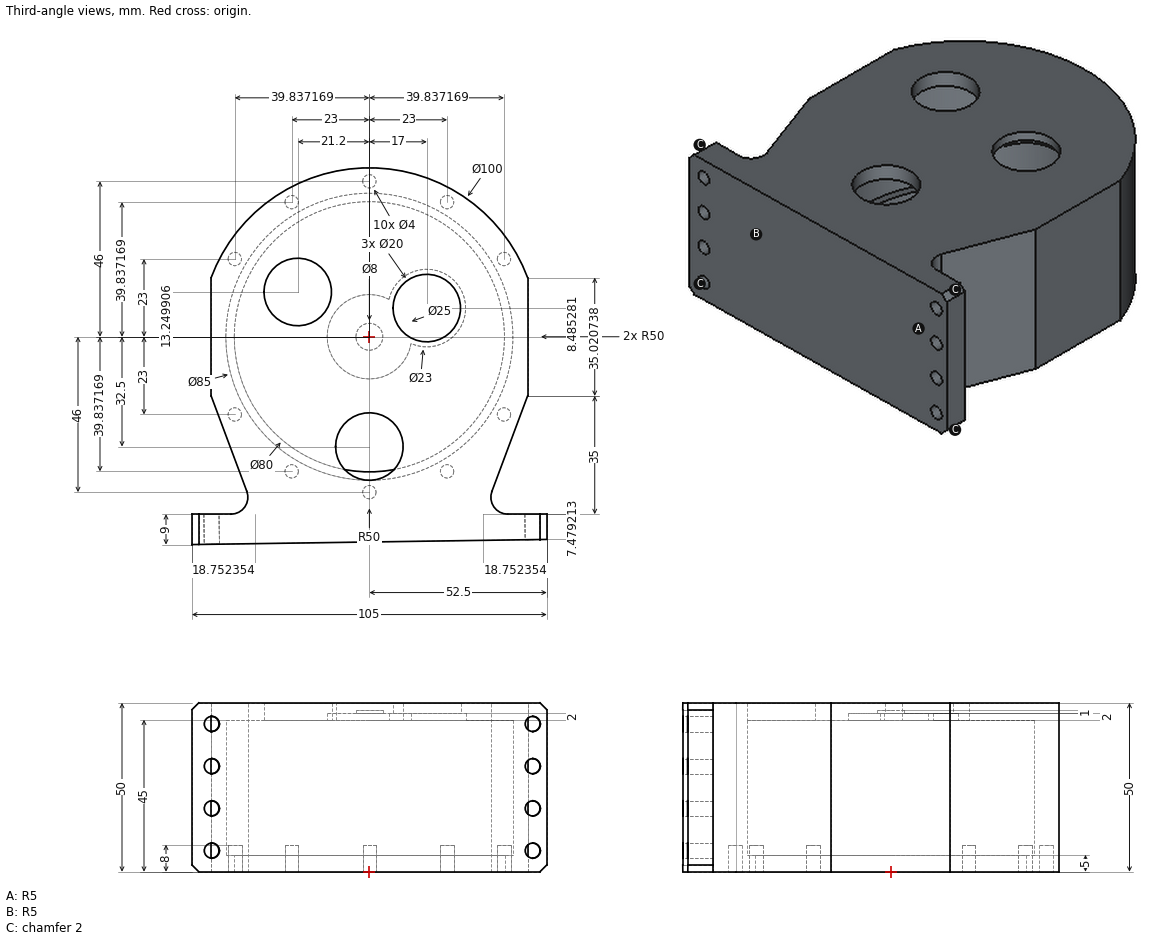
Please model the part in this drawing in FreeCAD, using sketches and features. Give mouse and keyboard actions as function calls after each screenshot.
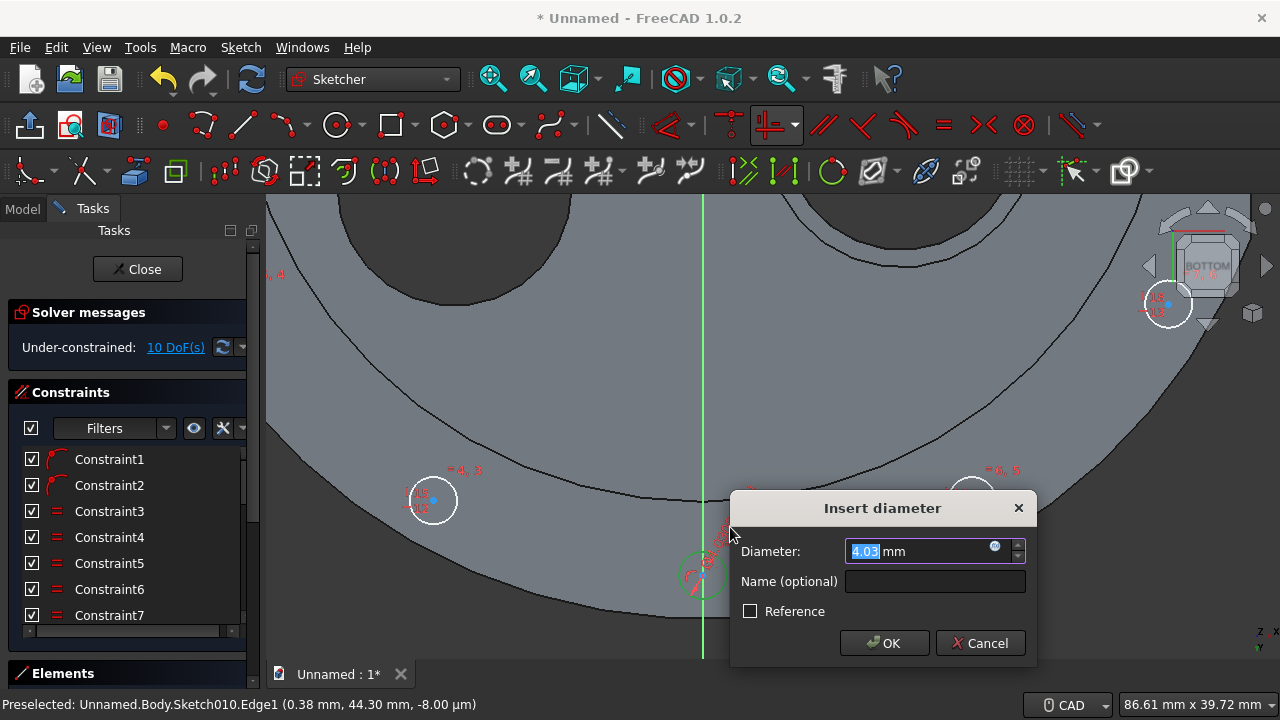
text(4)
key(Return)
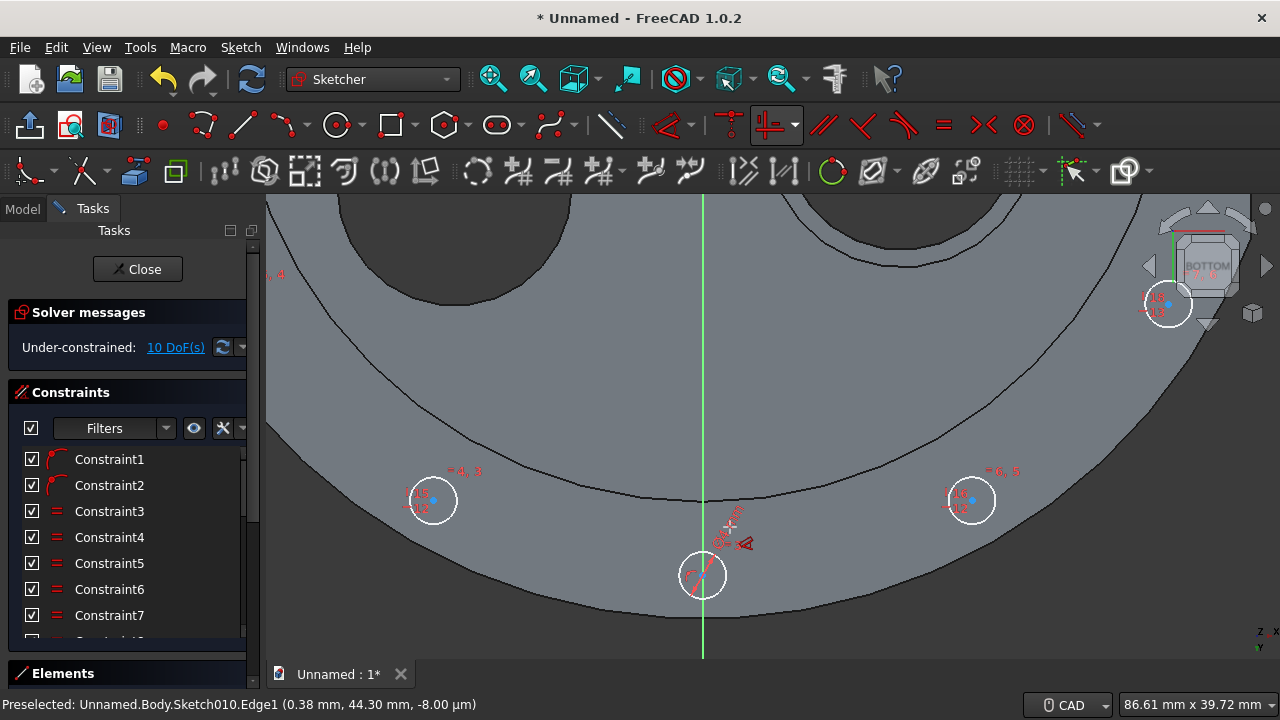
scroll(705, 555, down, 7)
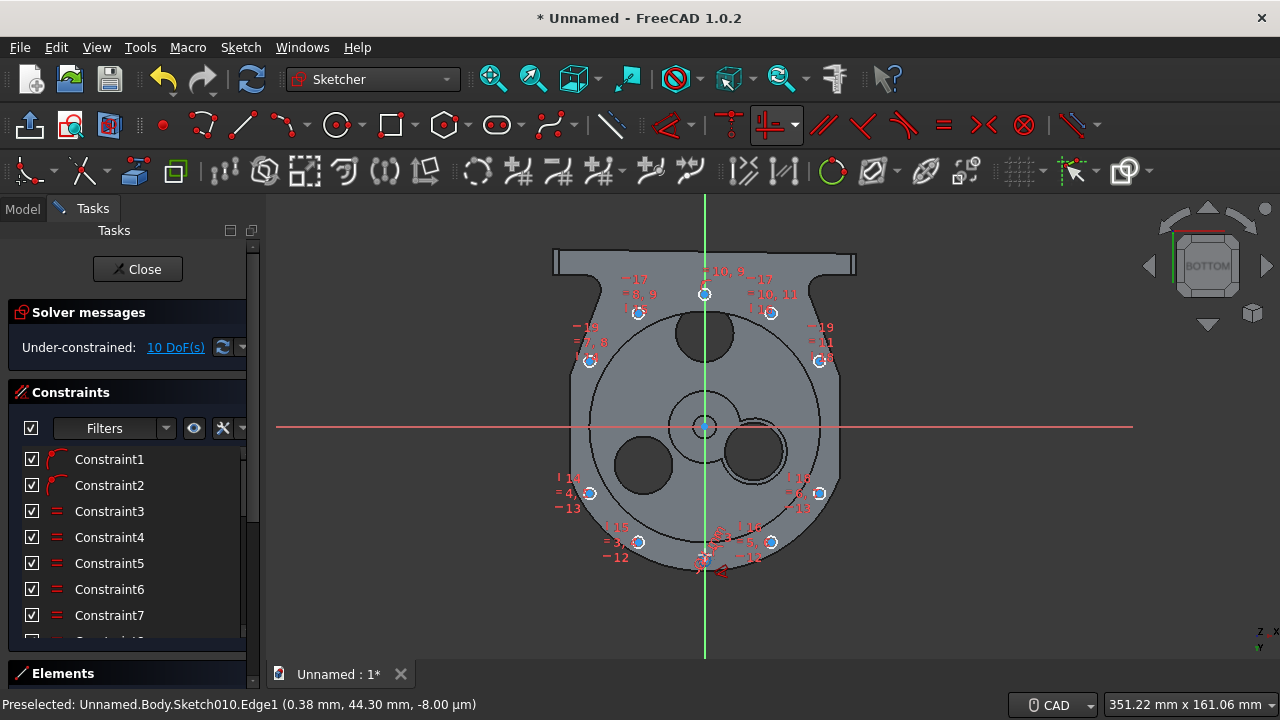
click(705, 561)
click(739, 494)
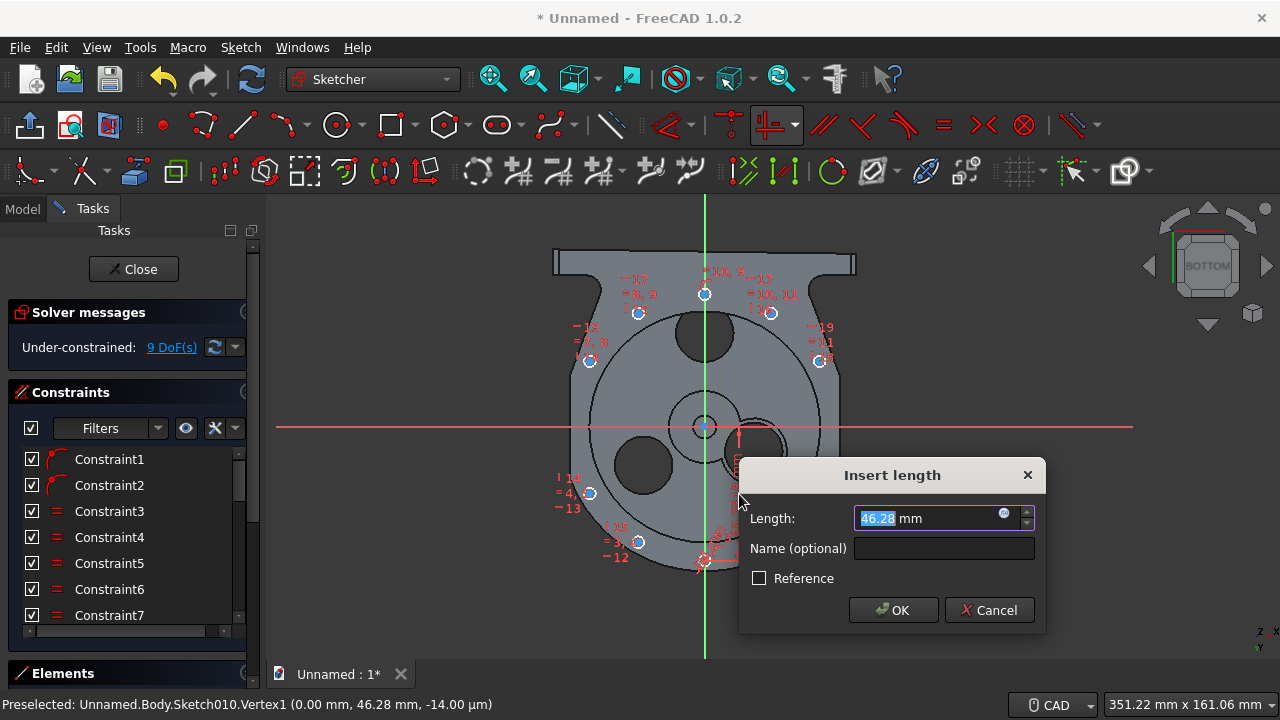
text(46)
key(Return)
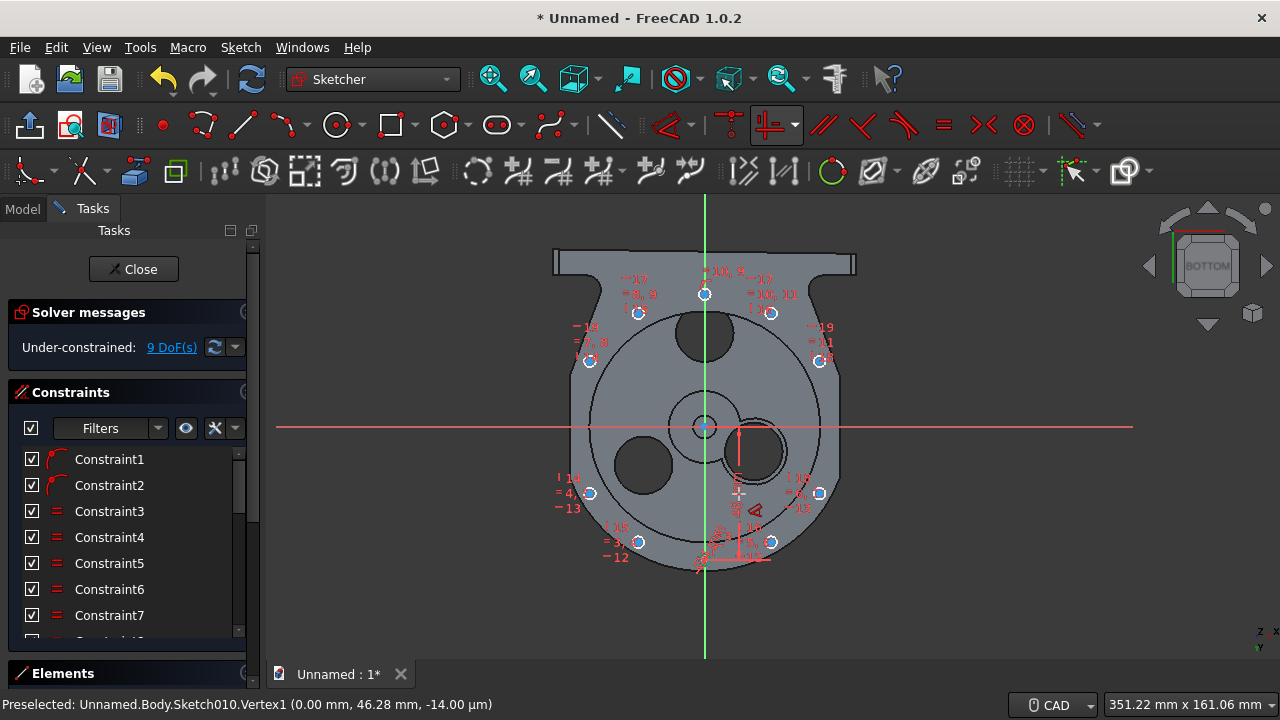
click(638, 542)
click(672, 576)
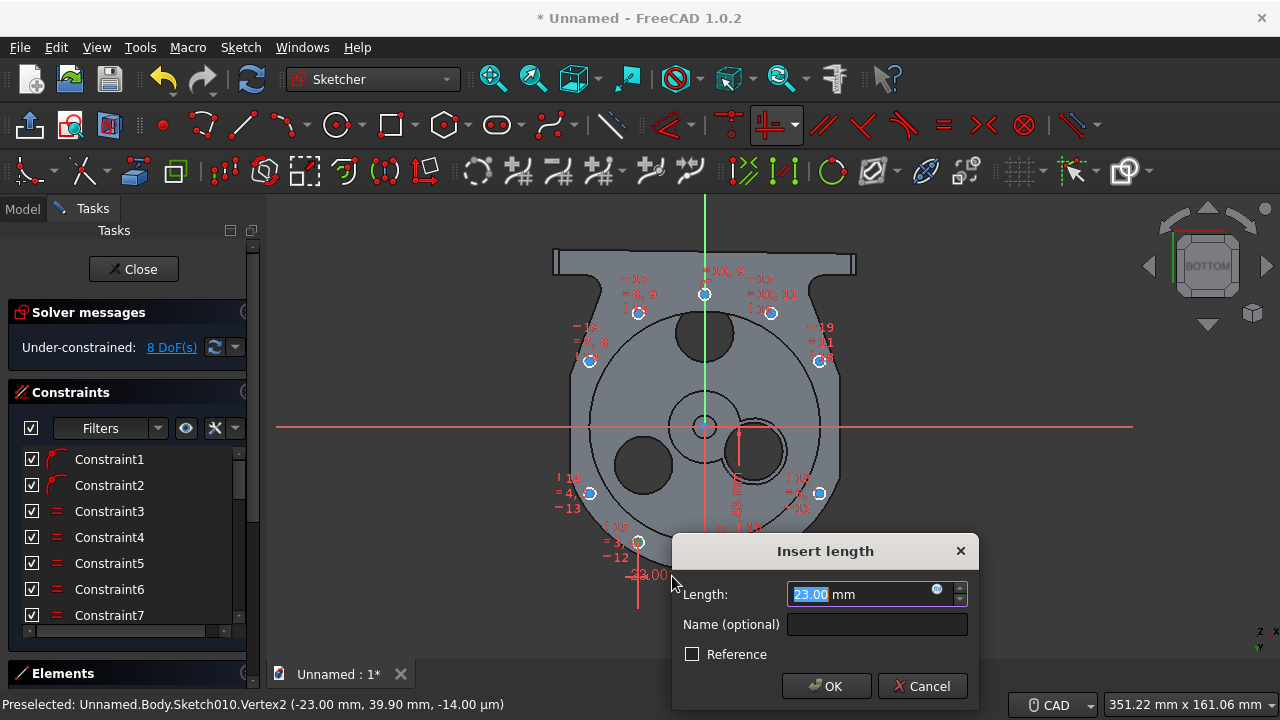
text(23)
key(Return)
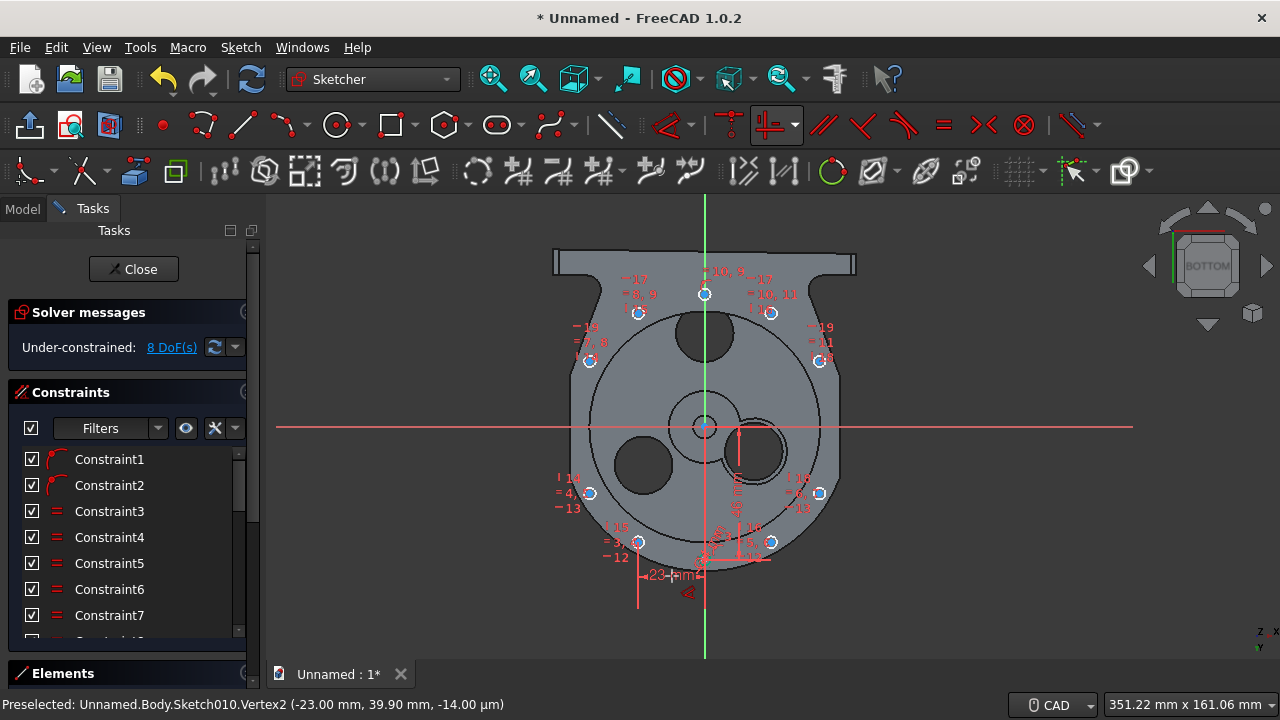
click(590, 494)
click(556, 460)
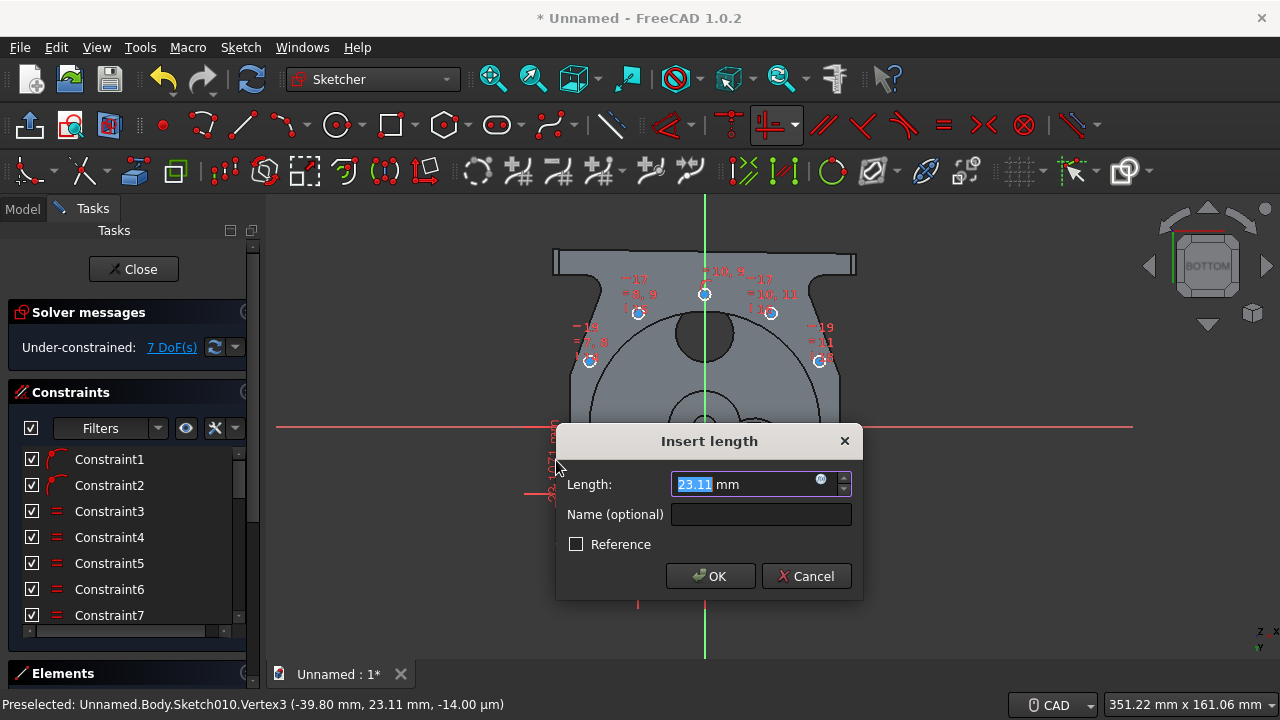
text(23)
key(Return)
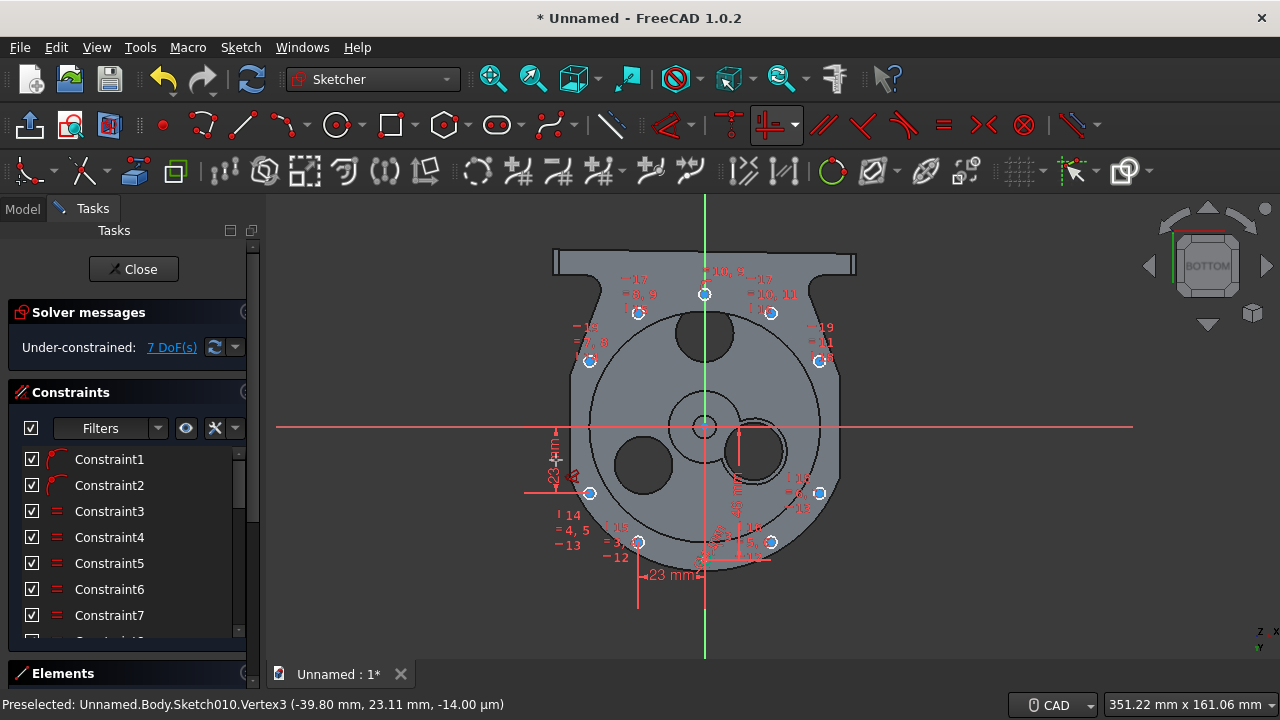
click(771, 542)
click(753, 576)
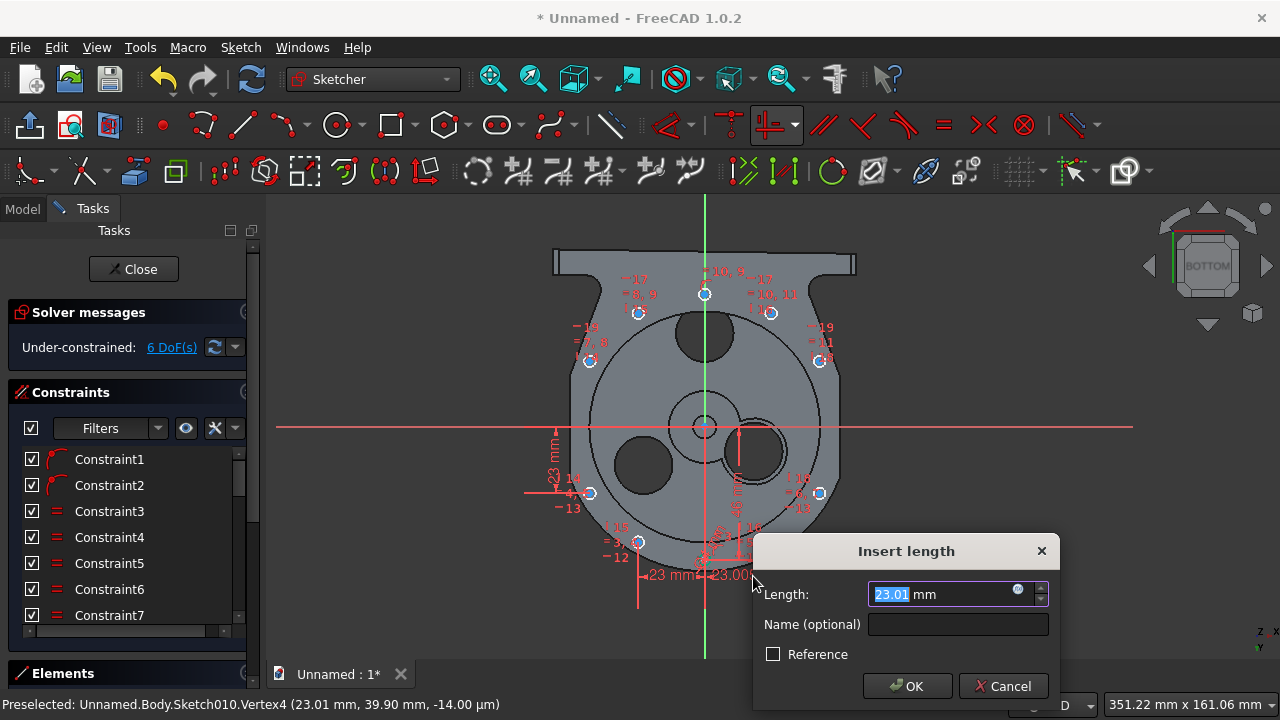
text(23)
key(Return)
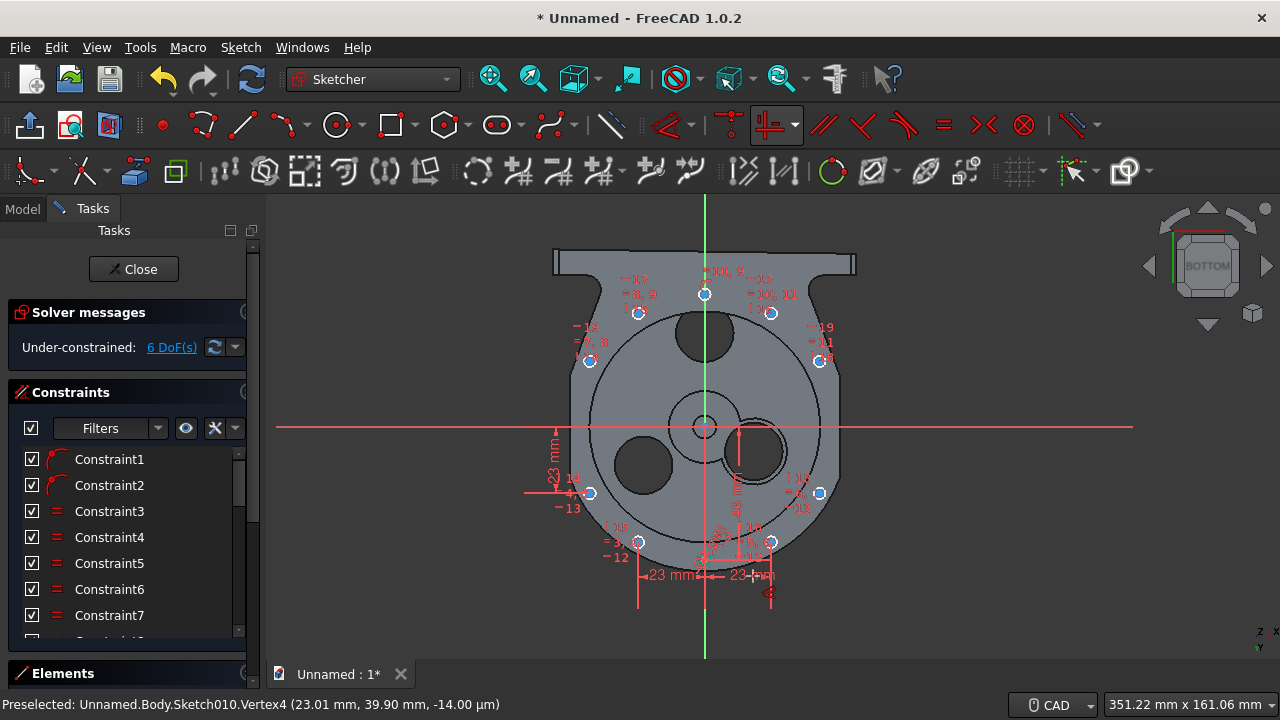
click(590, 361)
click(556, 394)